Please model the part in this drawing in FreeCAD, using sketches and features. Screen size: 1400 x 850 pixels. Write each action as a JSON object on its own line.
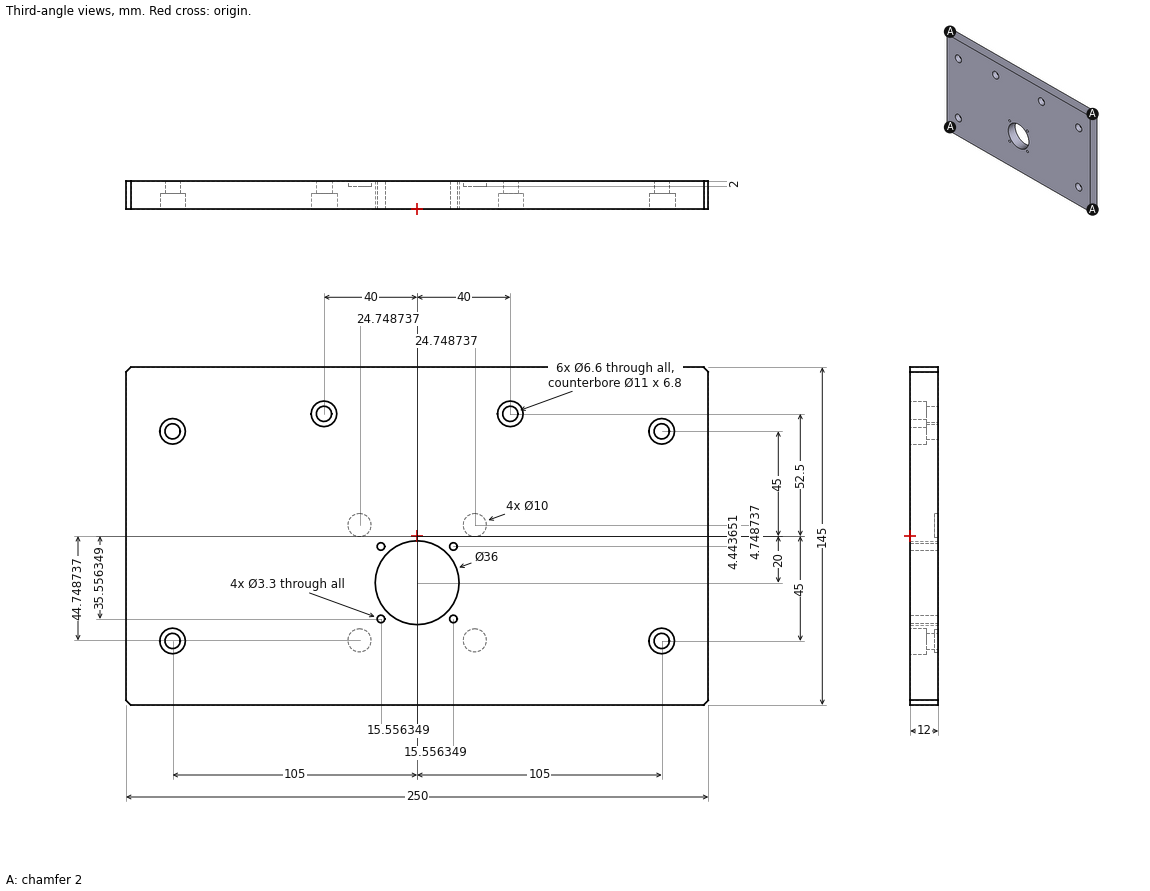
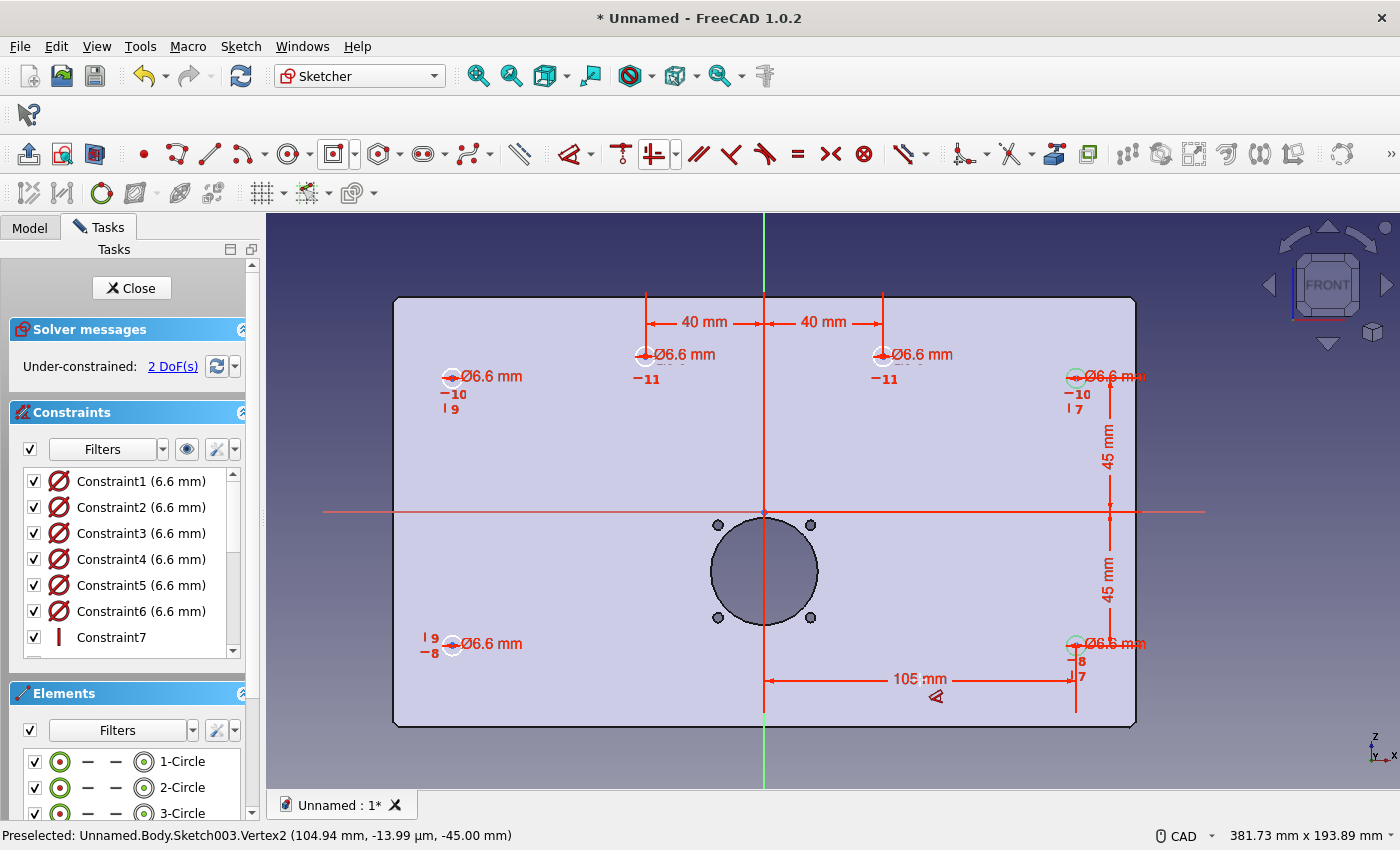
{"action": "left_click", "coordinate": [452, 646]}
{"action": "left_click", "coordinate": [608, 680]}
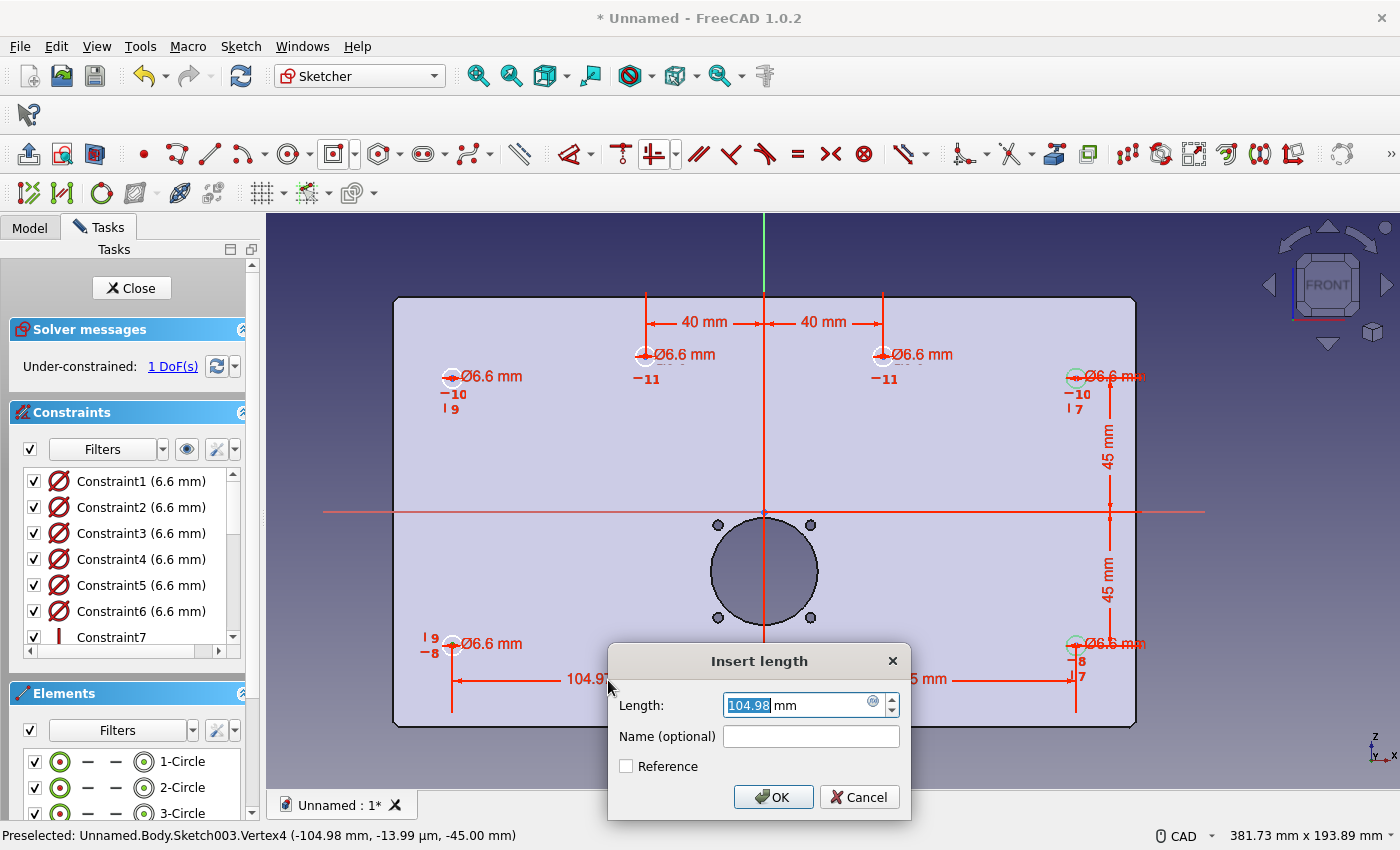
{"action": "type", "text": "105"}
{"action": "key", "text": "Return"}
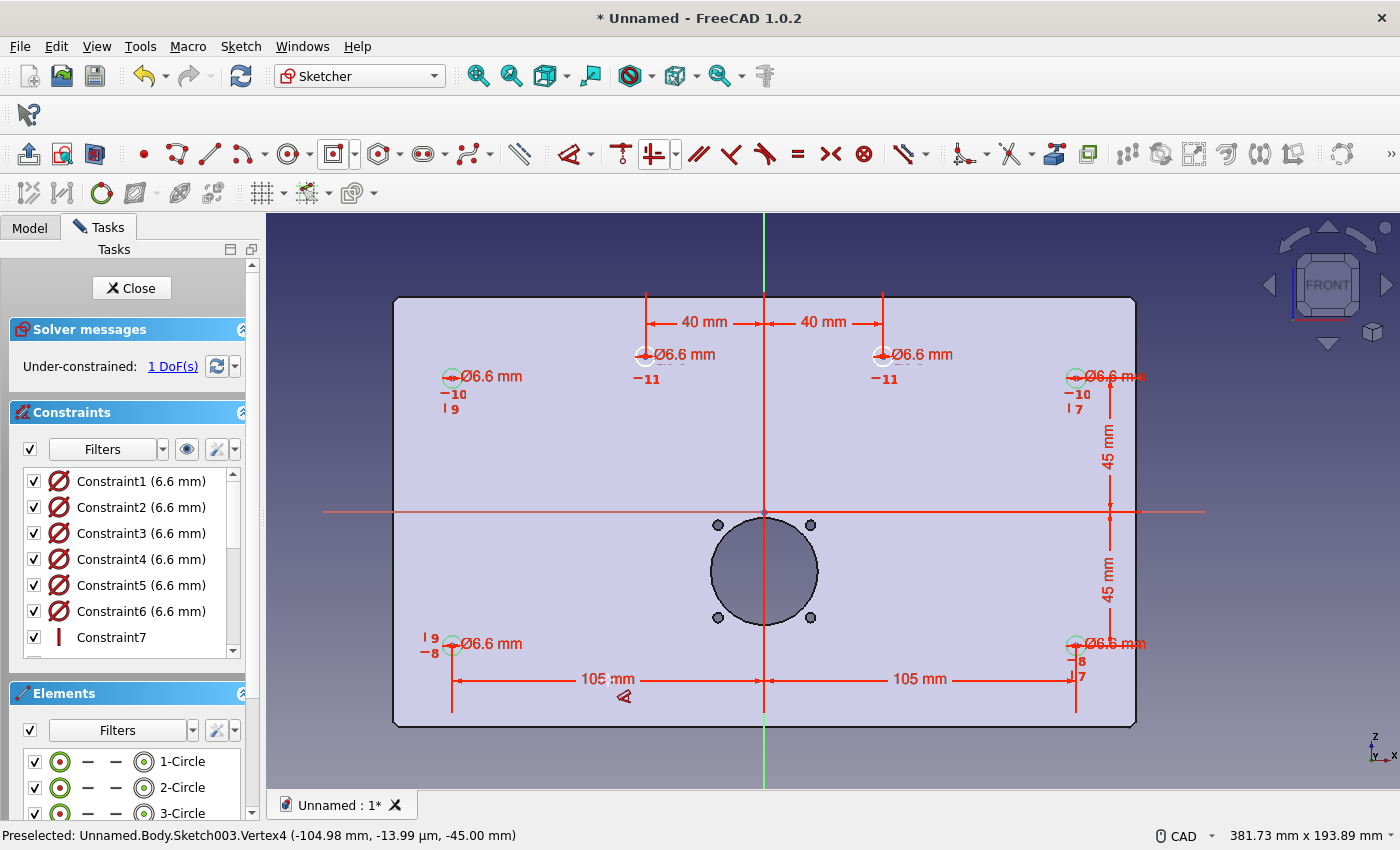
{"action": "left_click", "coordinate": [883, 357]}
{"action": "left_click", "coordinate": [917, 434]}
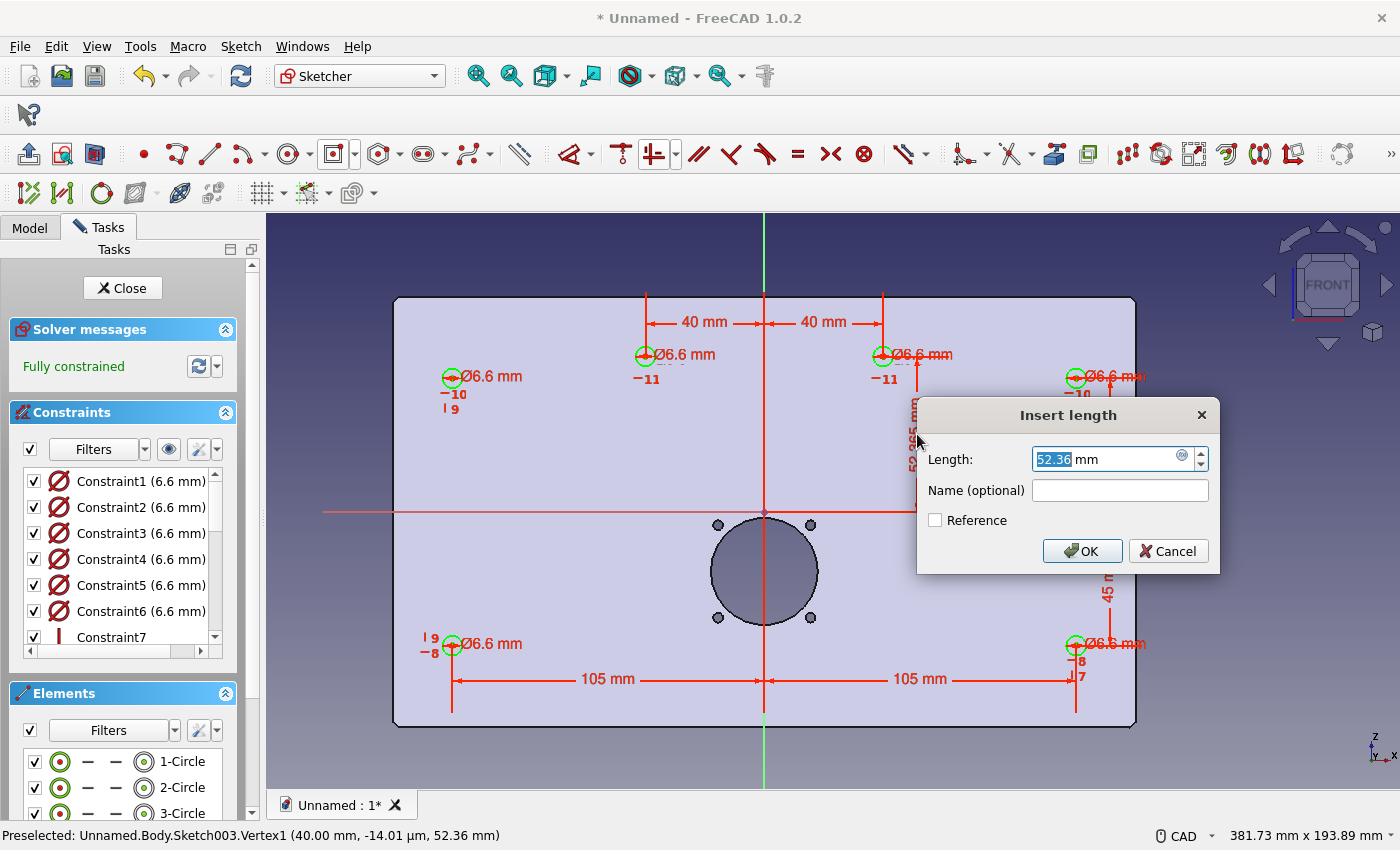
{"action": "type", "text": "52.5"}
{"action": "key", "text": "Return"}
{"action": "key", "text": "Escape"}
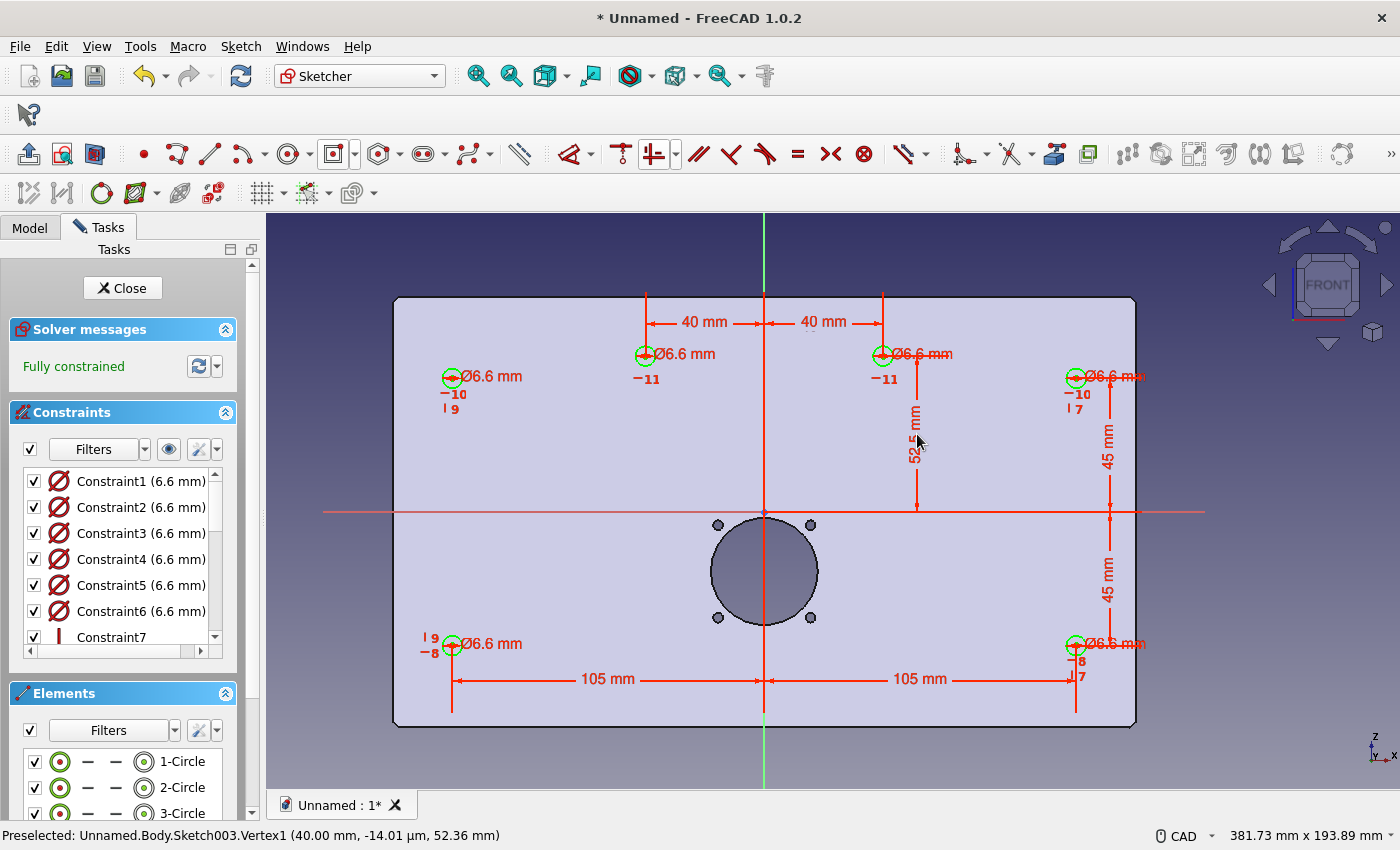
{"action": "left_click", "coordinate": [123, 288]}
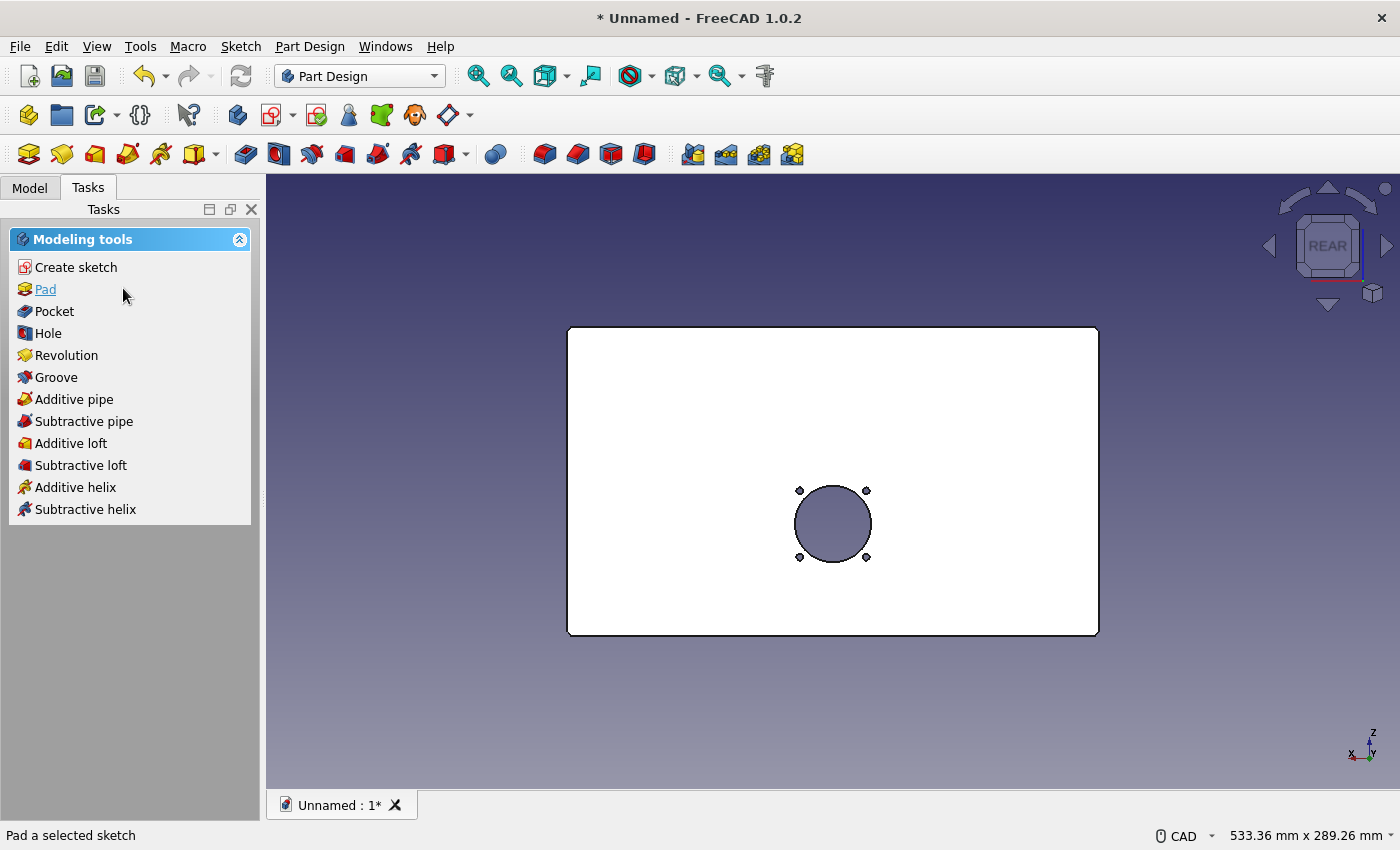
{"action": "left_click", "coordinate": [279, 154]}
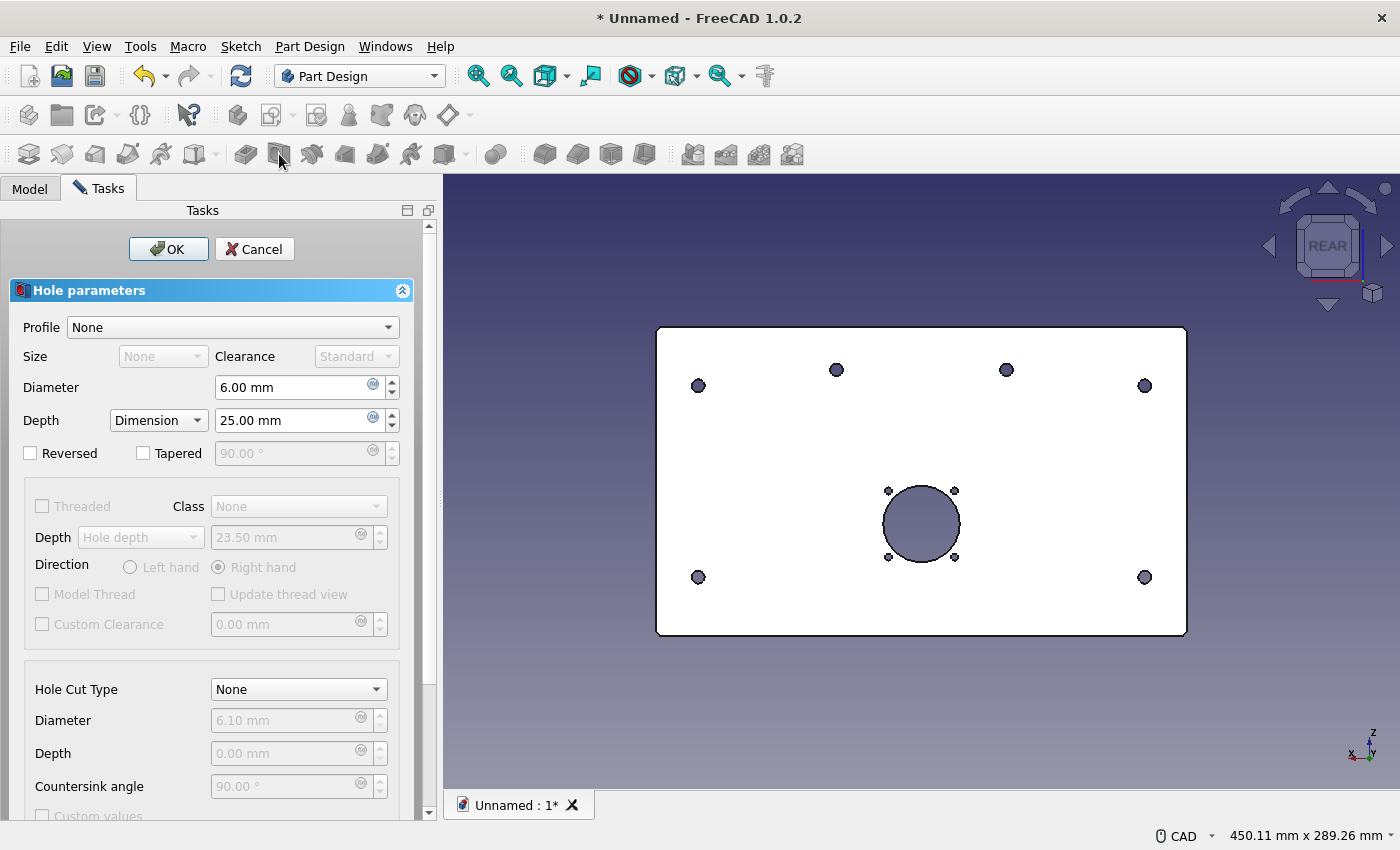
{"action": "triple_click", "coordinate": [300, 388]}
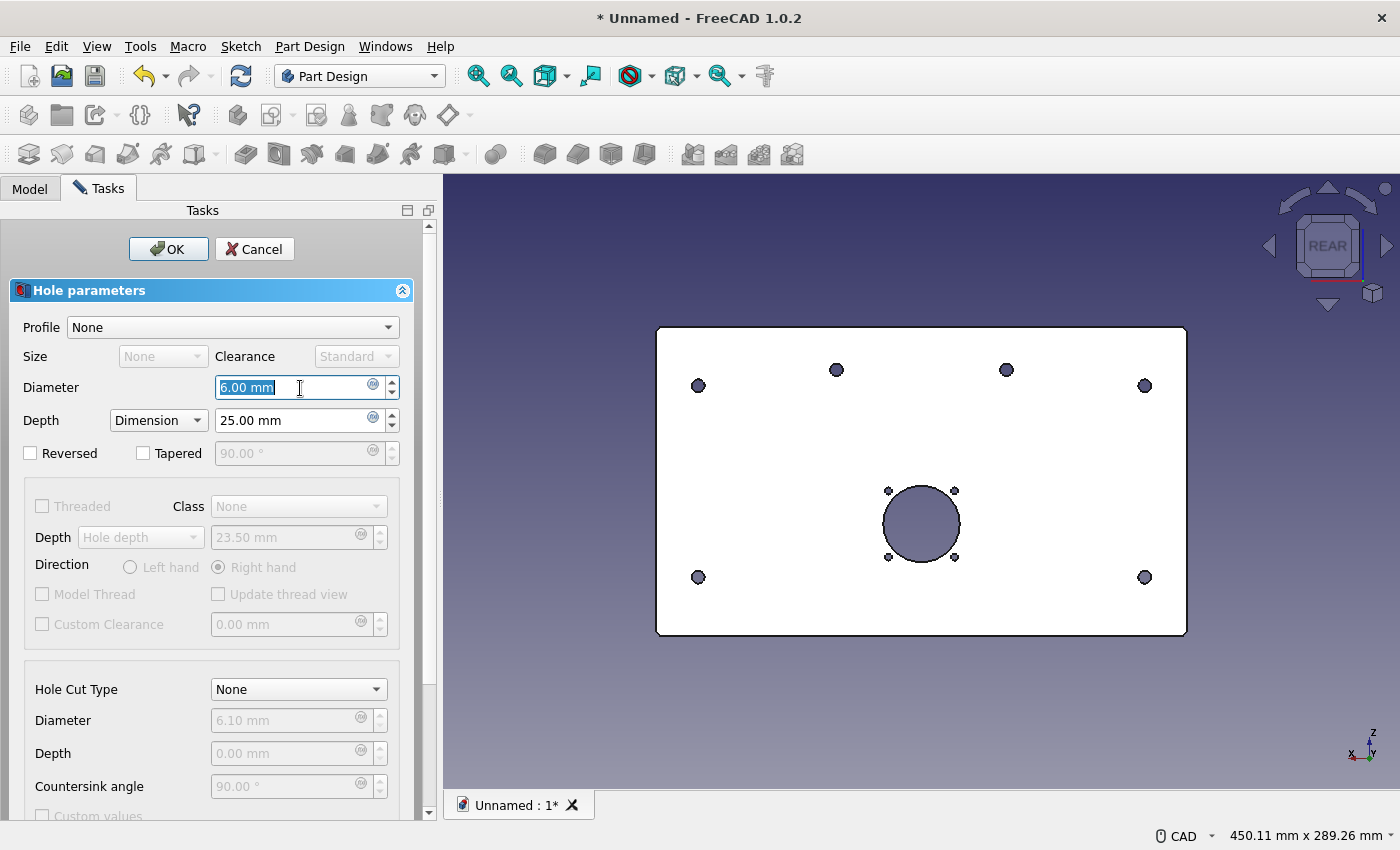
{"action": "type", "text": "6.6"}
{"action": "key", "text": "Tab"}